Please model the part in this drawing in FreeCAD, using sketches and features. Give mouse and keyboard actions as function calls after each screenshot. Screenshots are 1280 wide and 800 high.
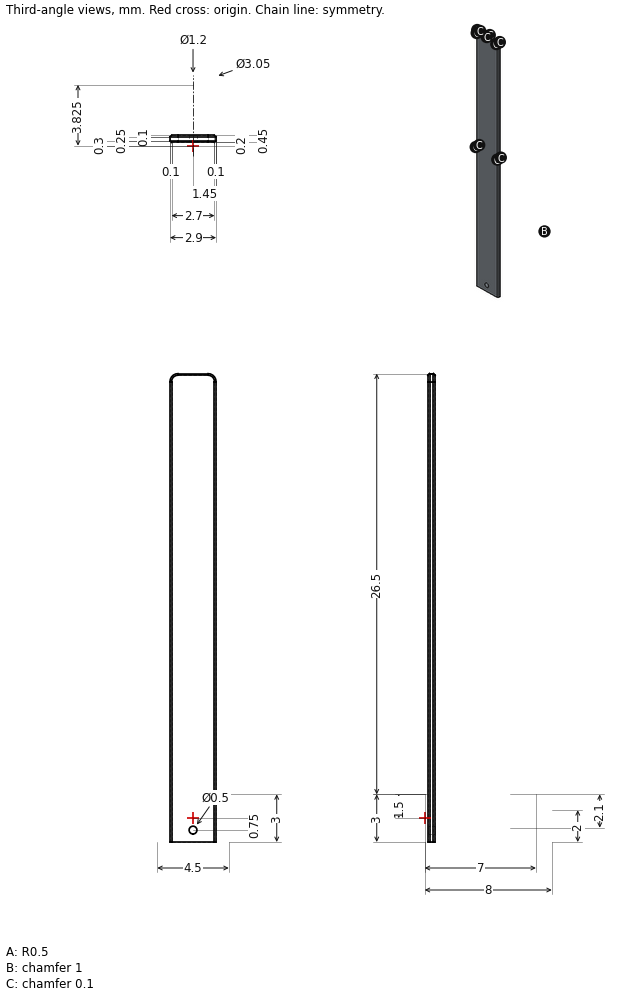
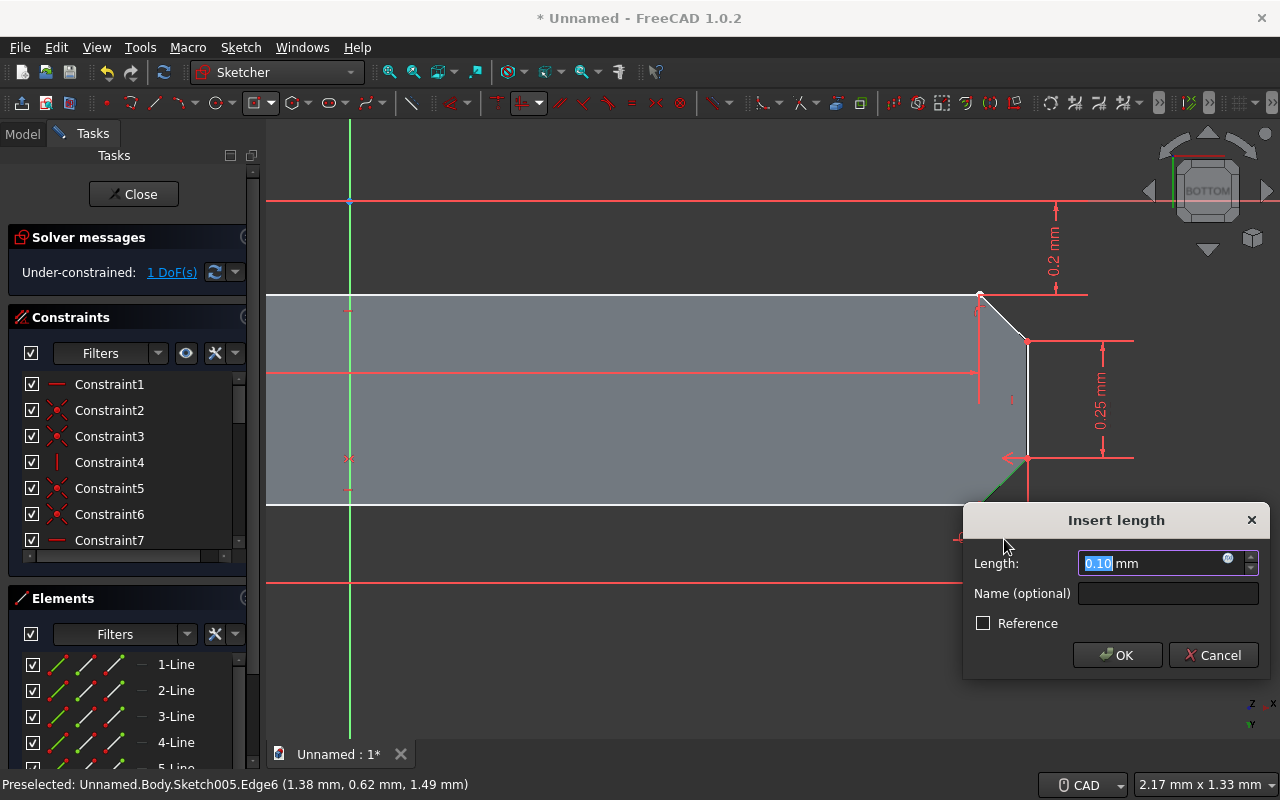
text(0.1)
key(Return)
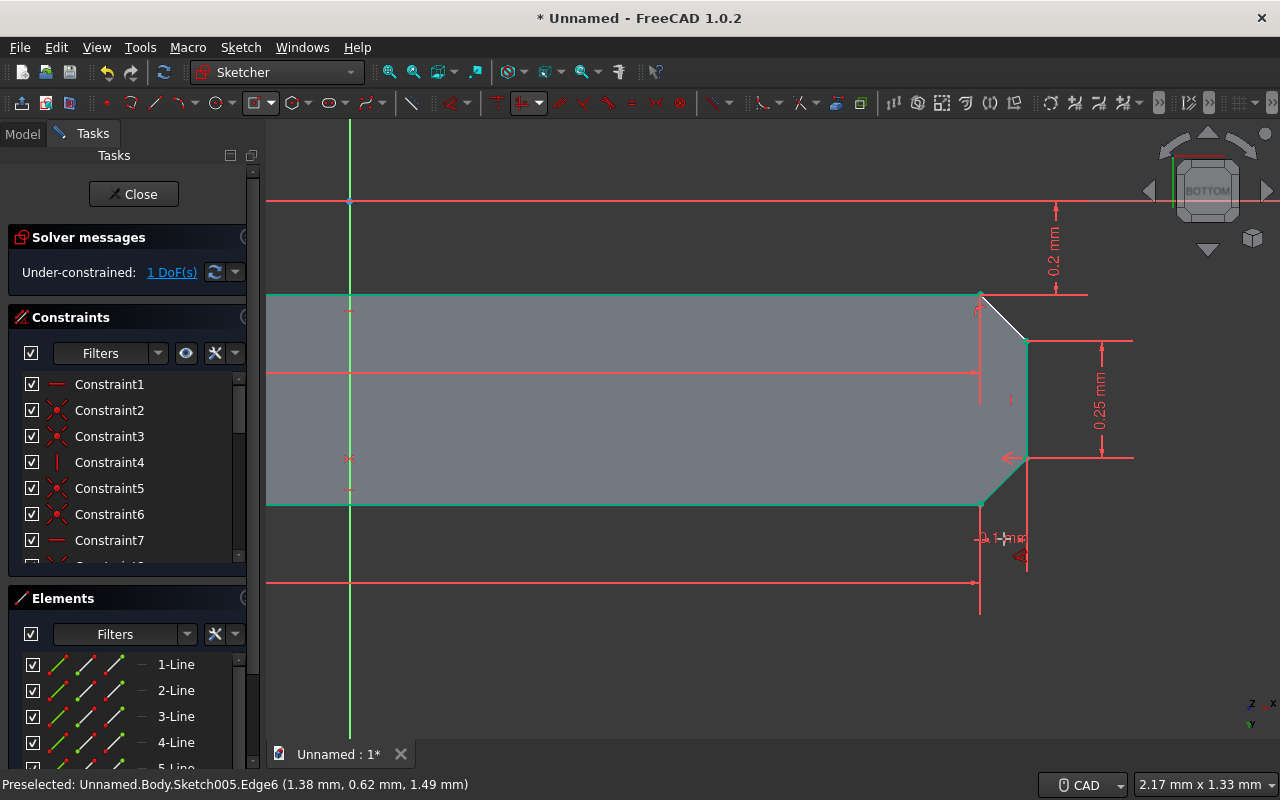
click(1013, 327)
click(1004, 375)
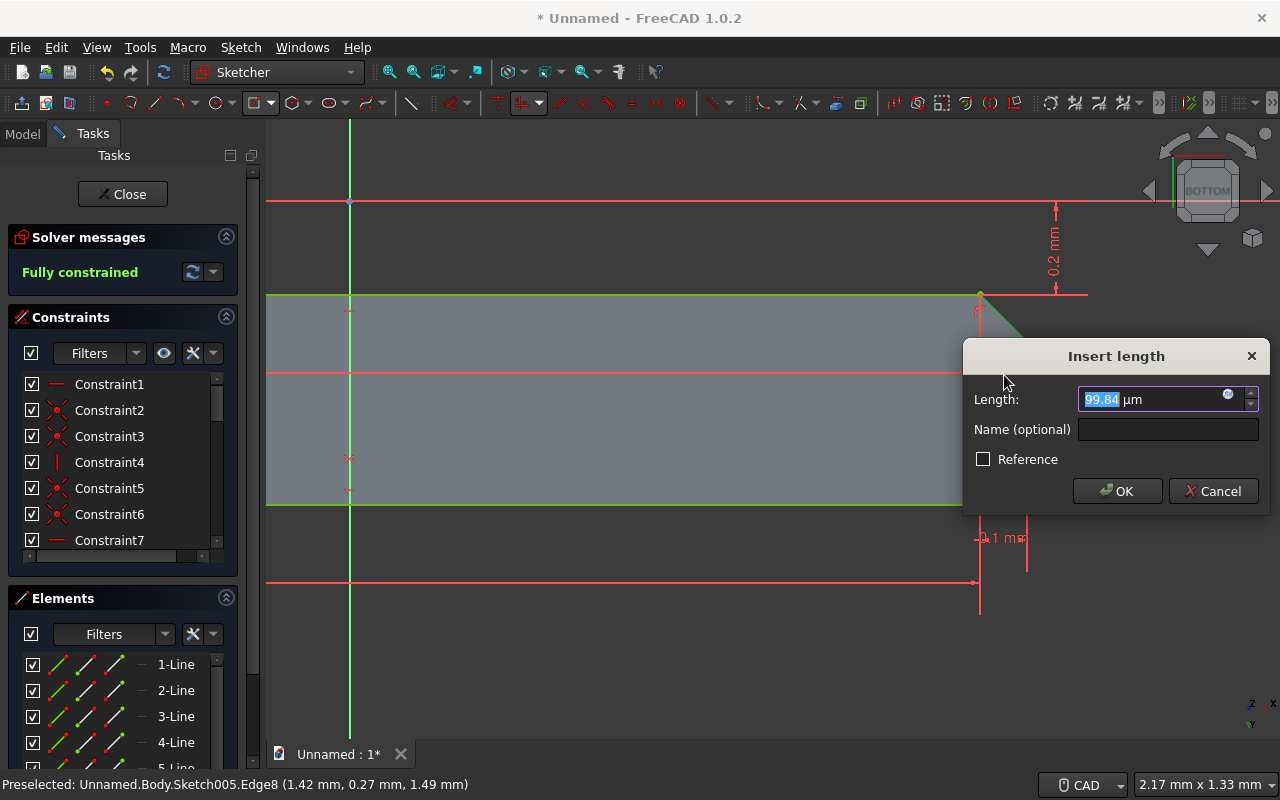
key(ctrl+a)
text(0.1 mm)
key(Return)
key(Escape)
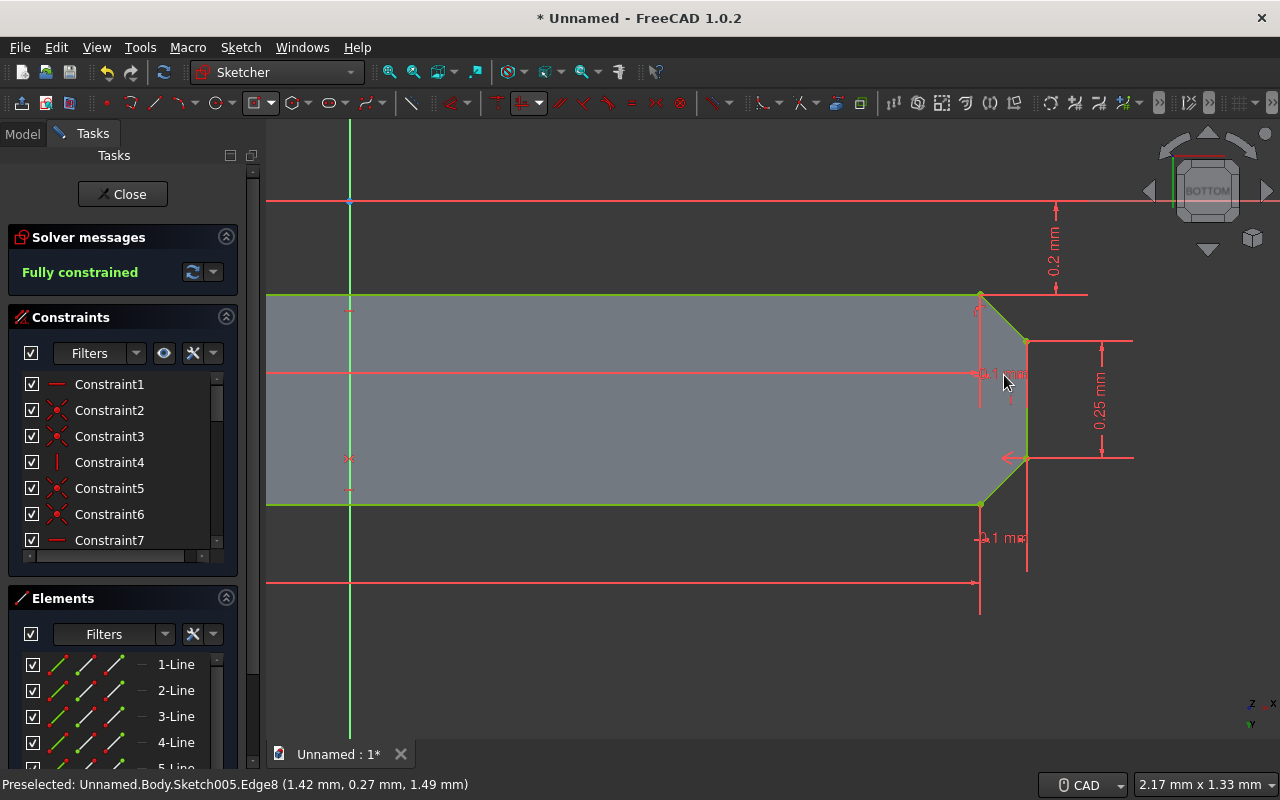
click(123, 194)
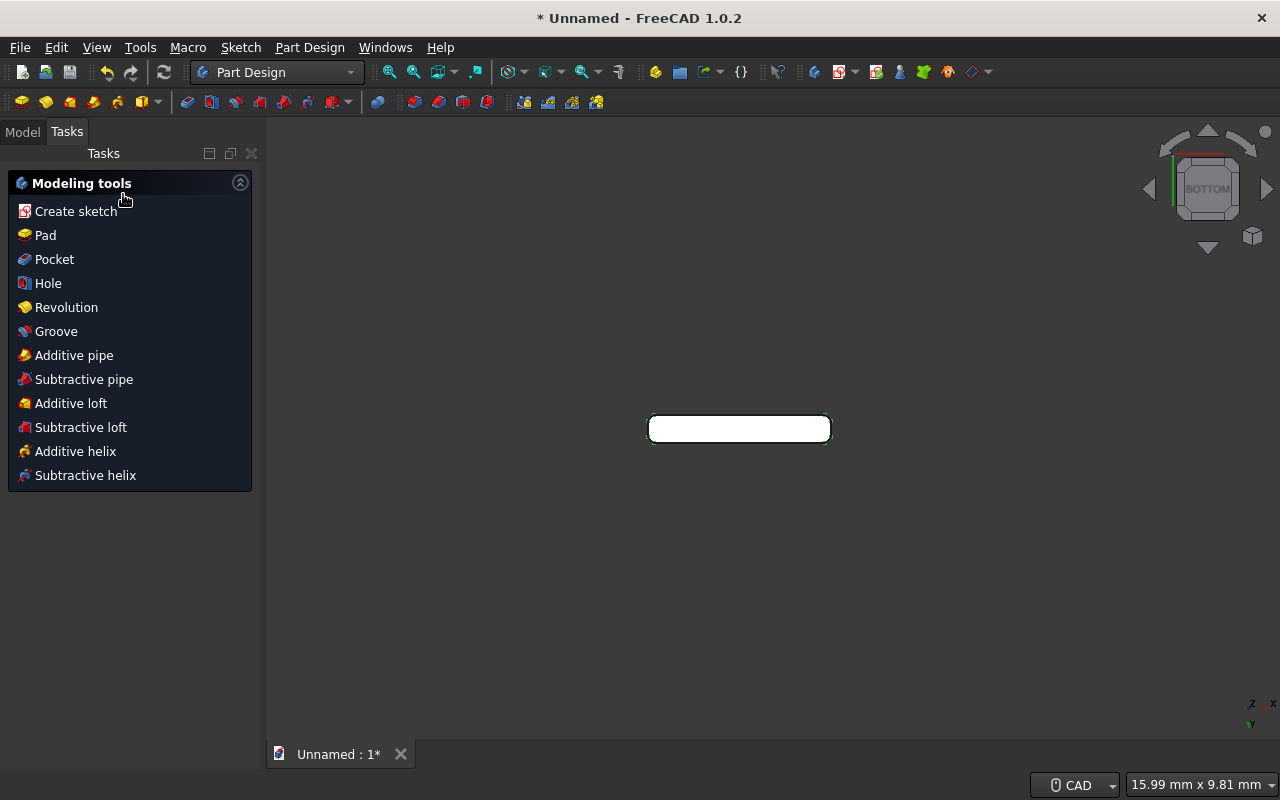
click(22, 102)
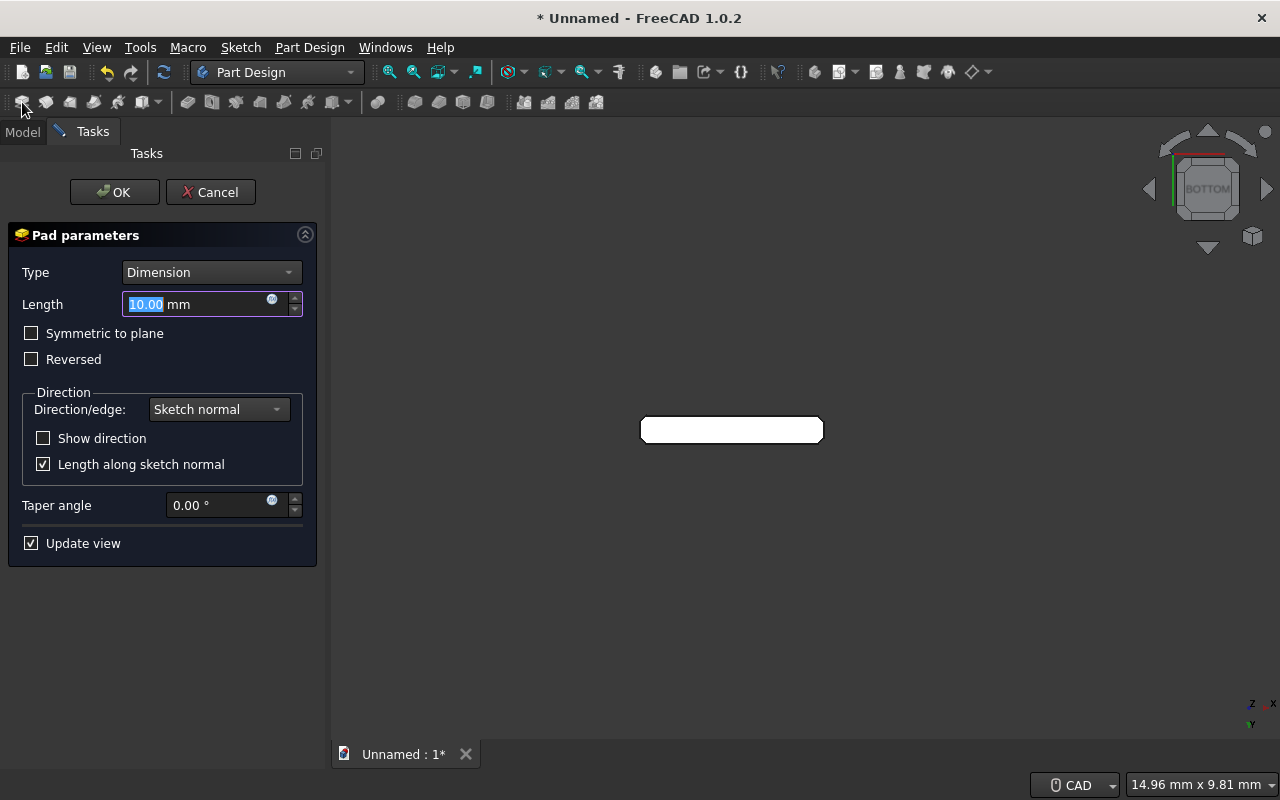
text(3)
key(Tab)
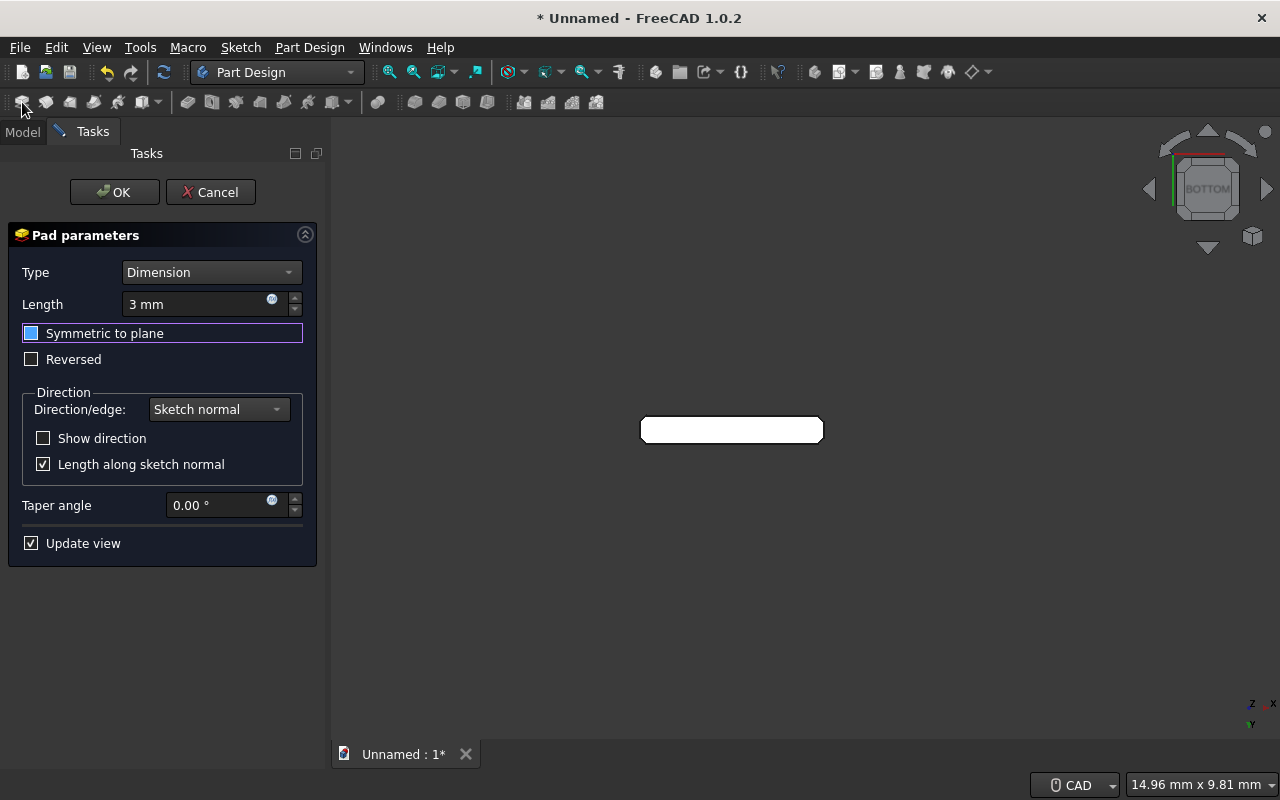
click(115, 192)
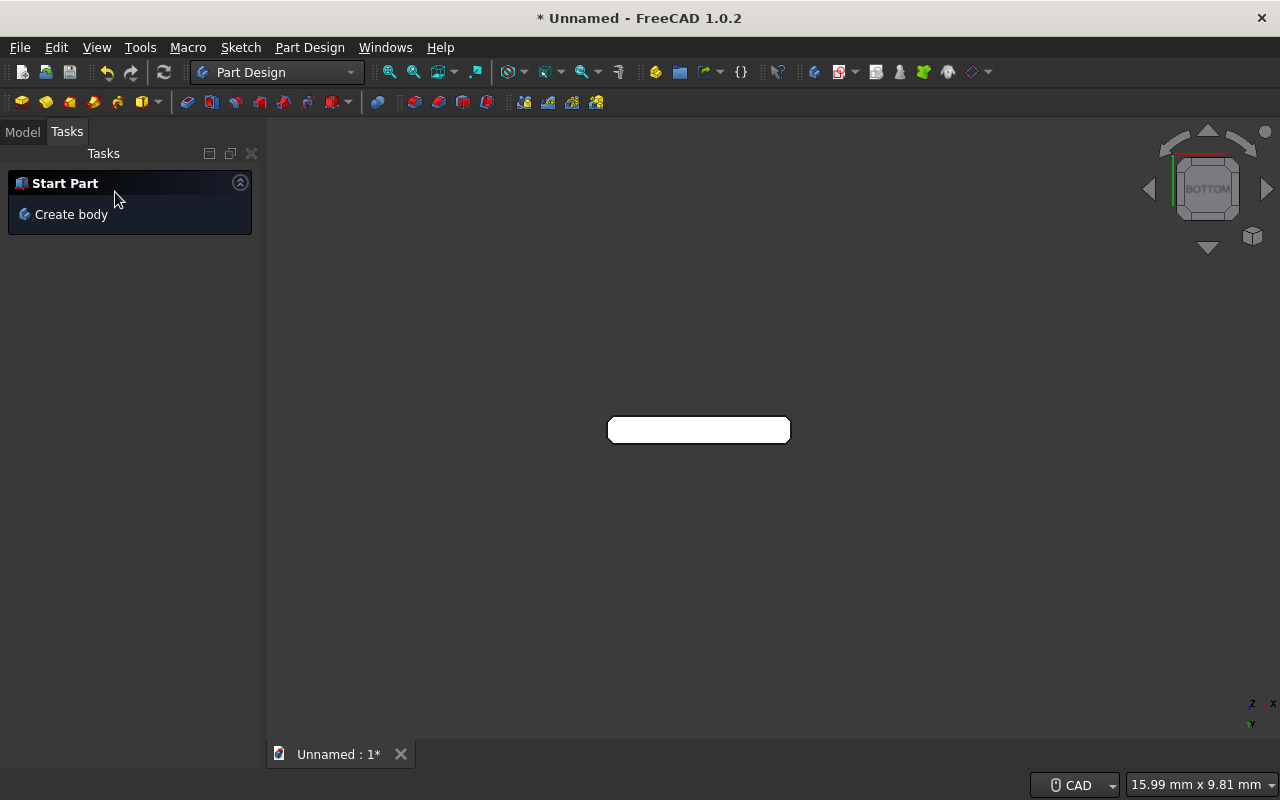
key(v)
key(f)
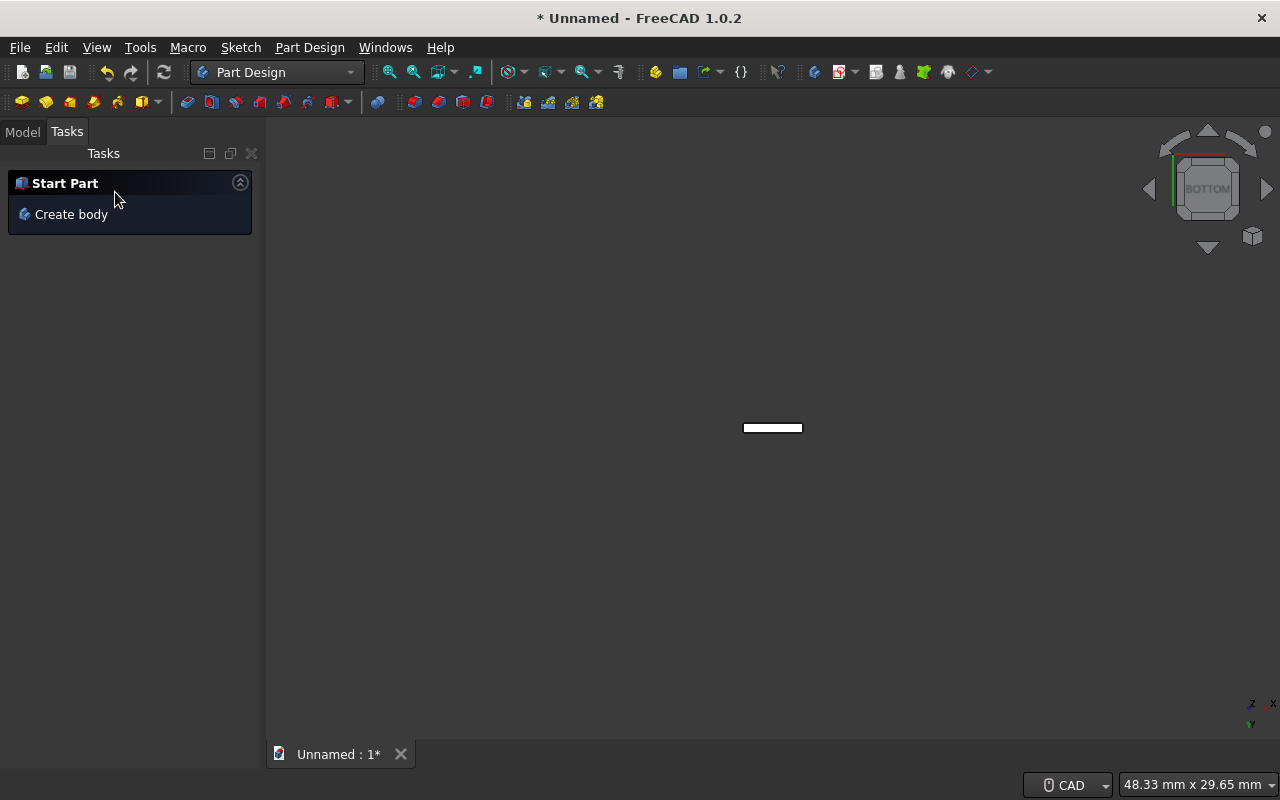
key(0)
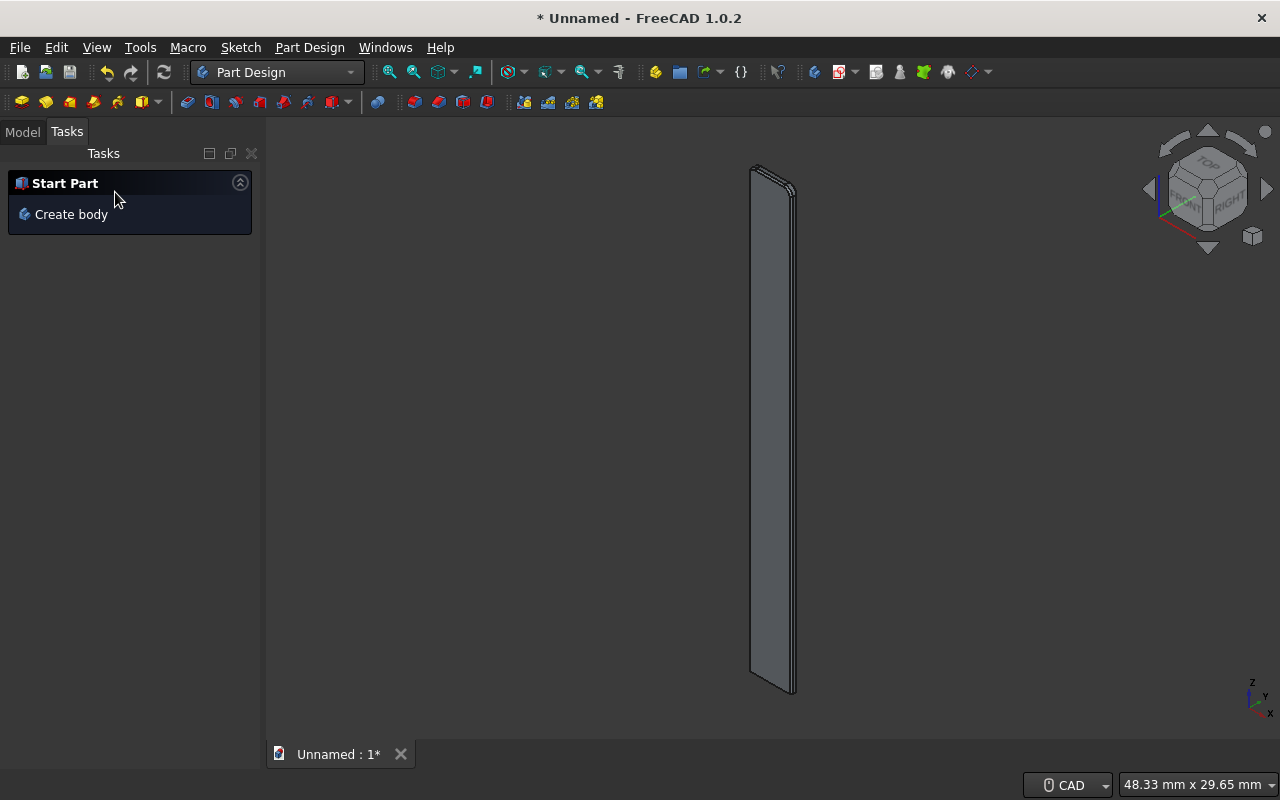
click(770, 214)